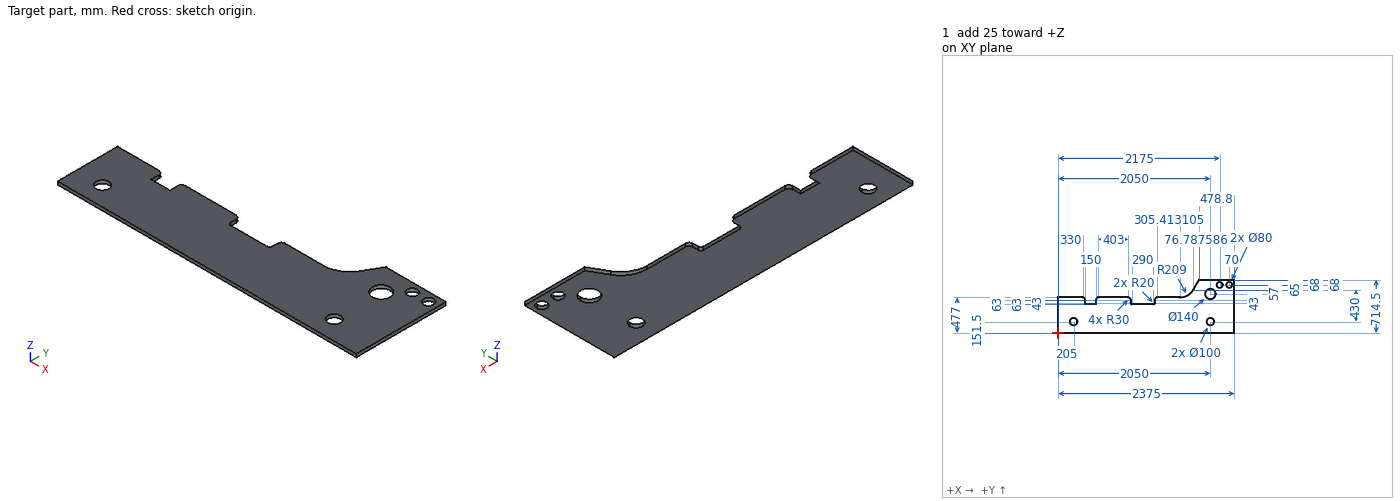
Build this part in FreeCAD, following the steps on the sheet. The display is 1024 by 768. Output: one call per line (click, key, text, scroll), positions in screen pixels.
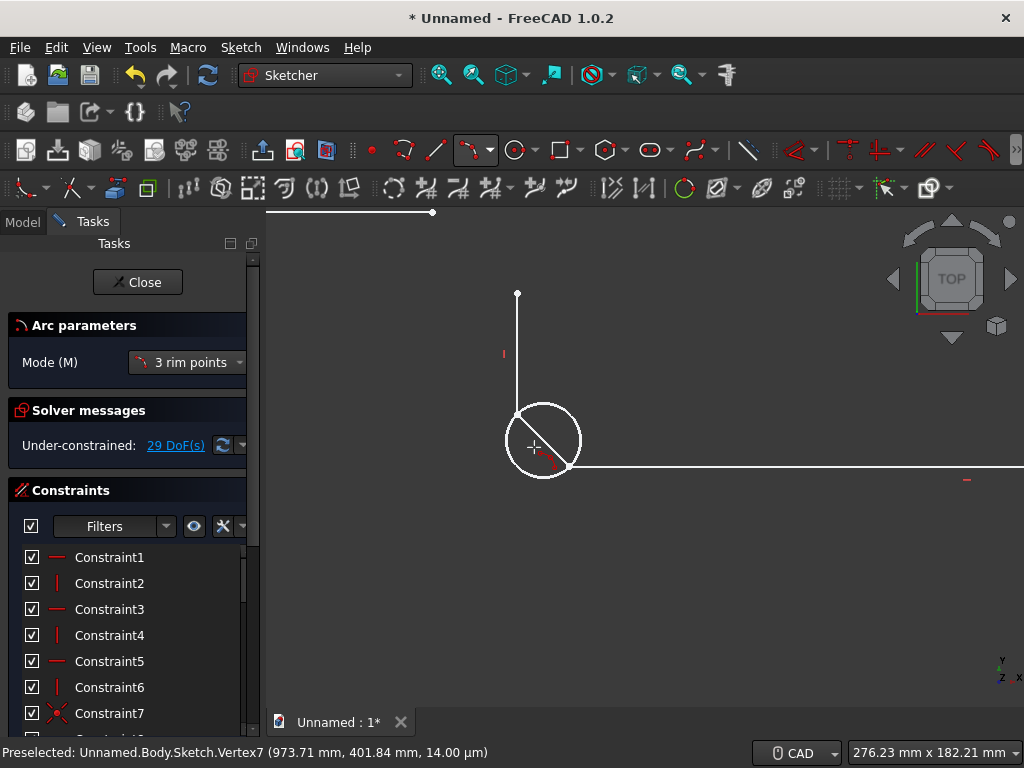
click(531, 447)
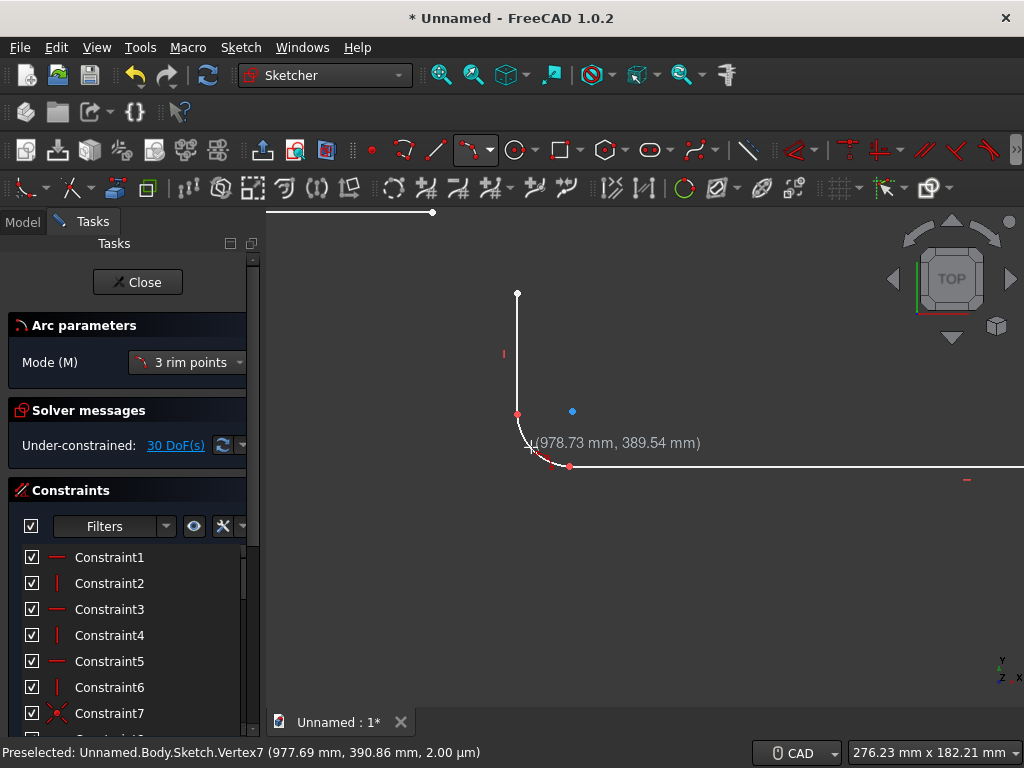
scroll(542, 452, down, 14)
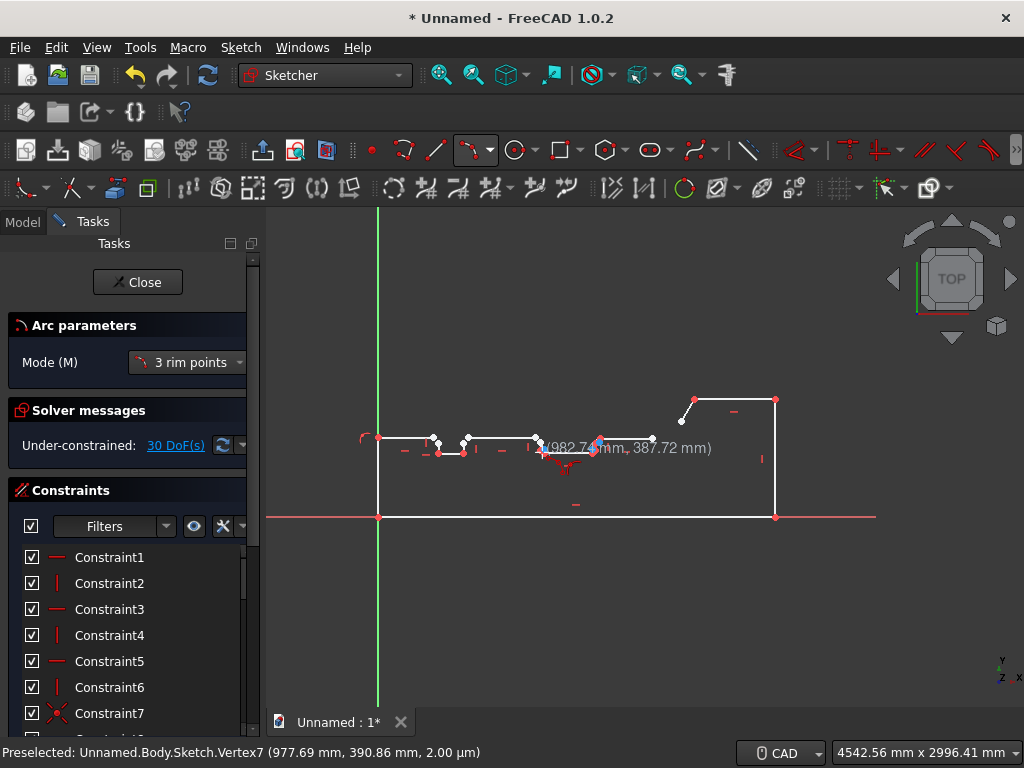
scroll(541, 443, up, 8)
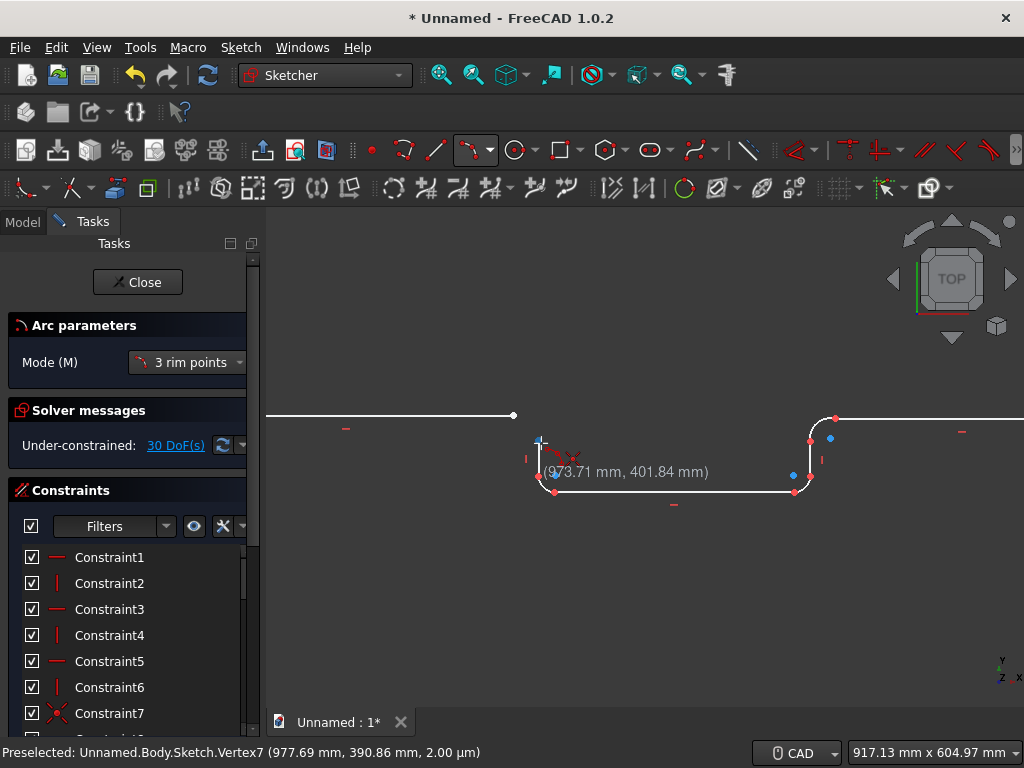
click(539, 440)
click(513, 416)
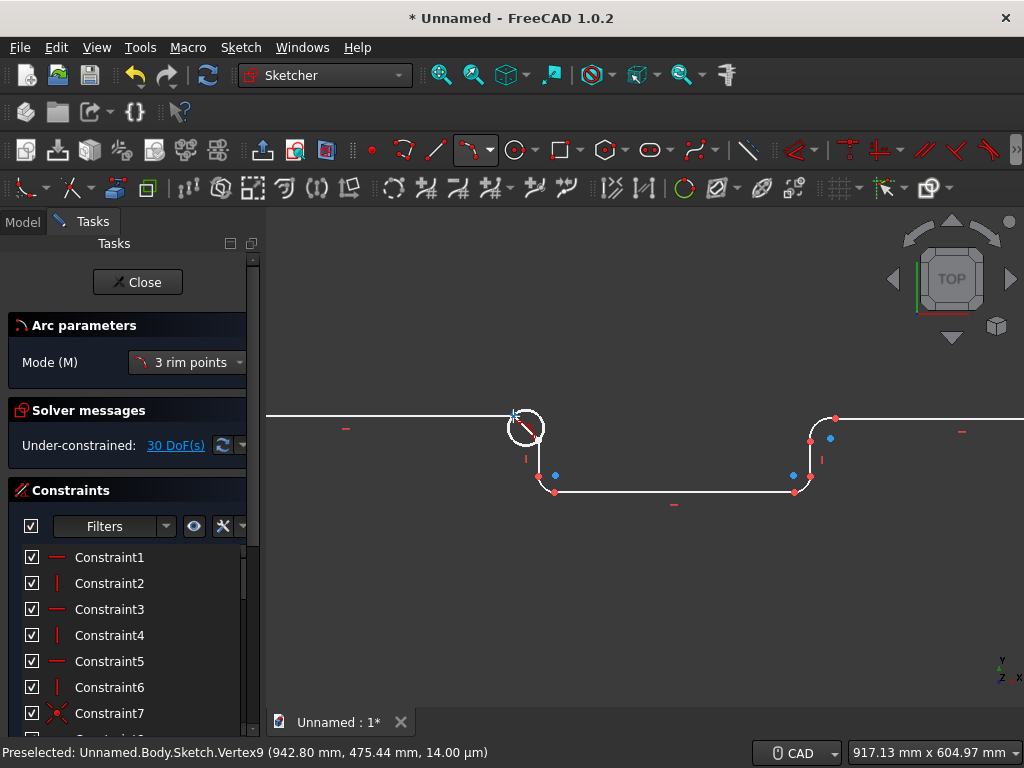
scroll(531, 422, up, 4)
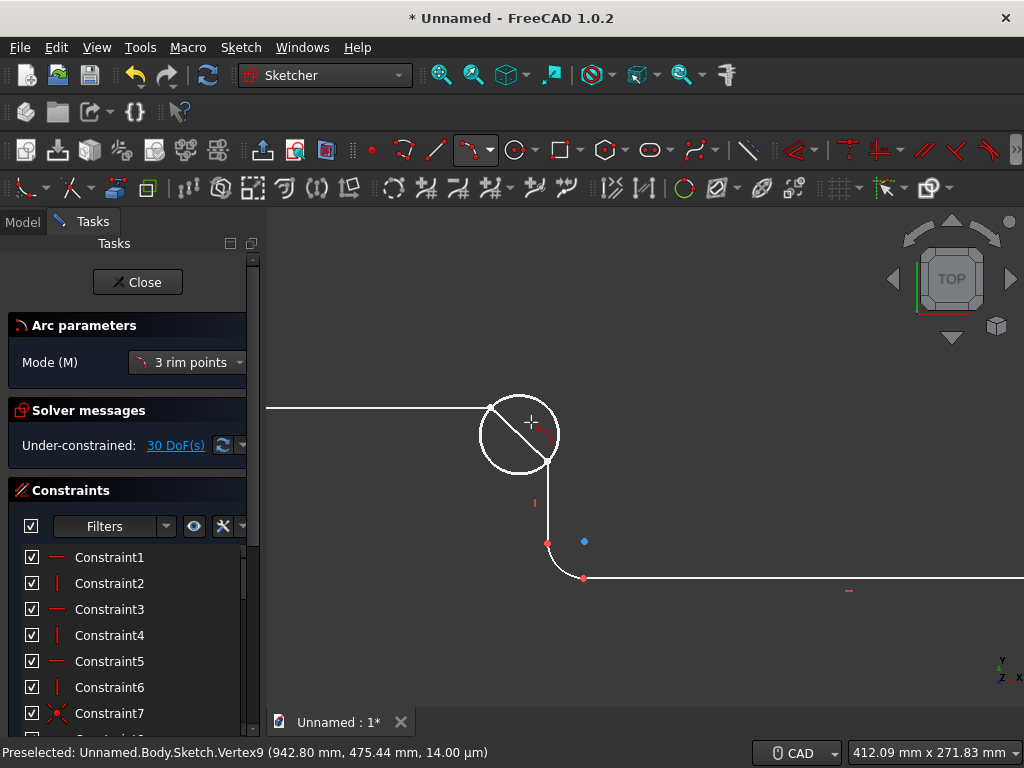
click(530, 421)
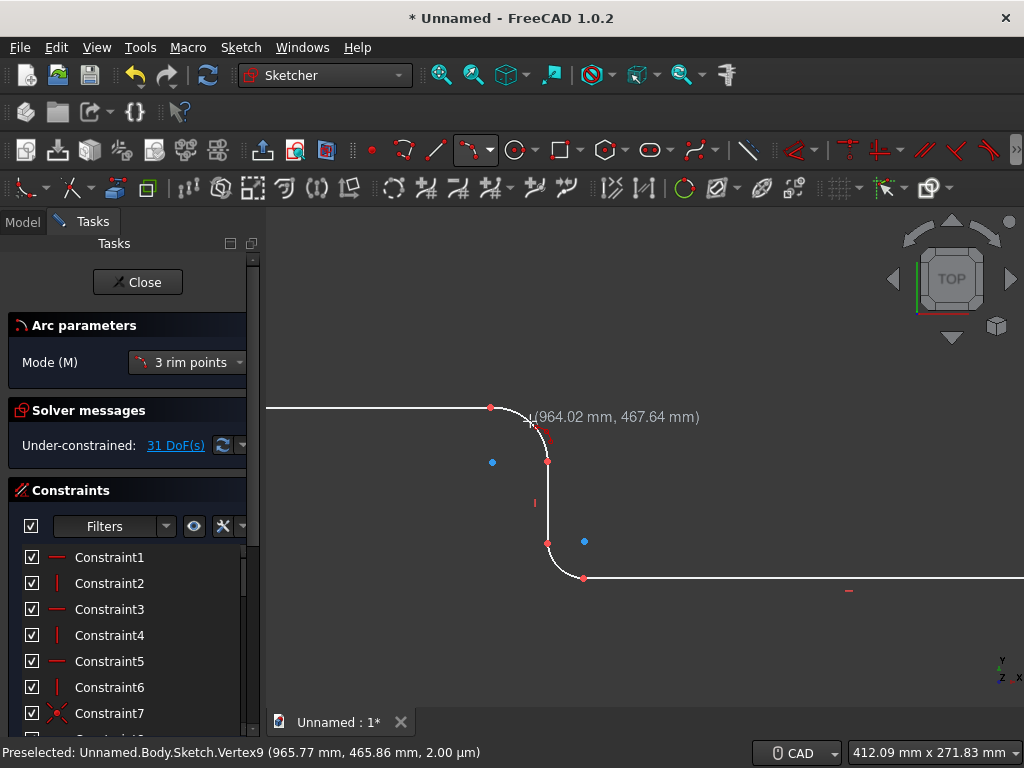
scroll(540, 440, down, 12)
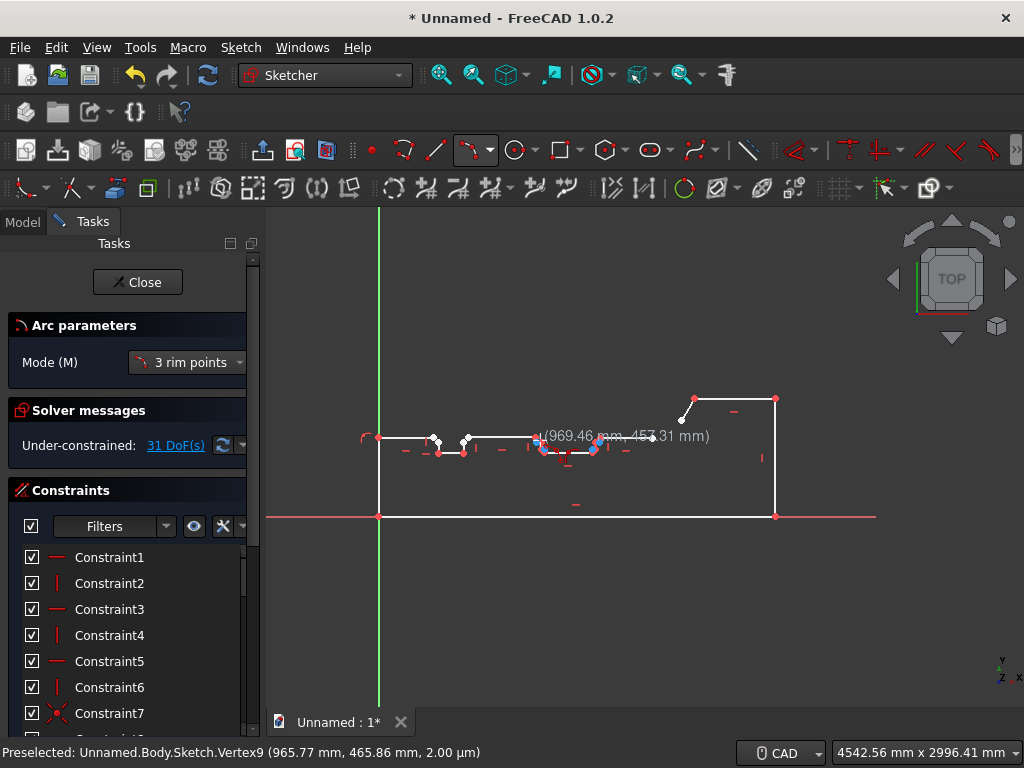
scroll(469, 437, up, 5)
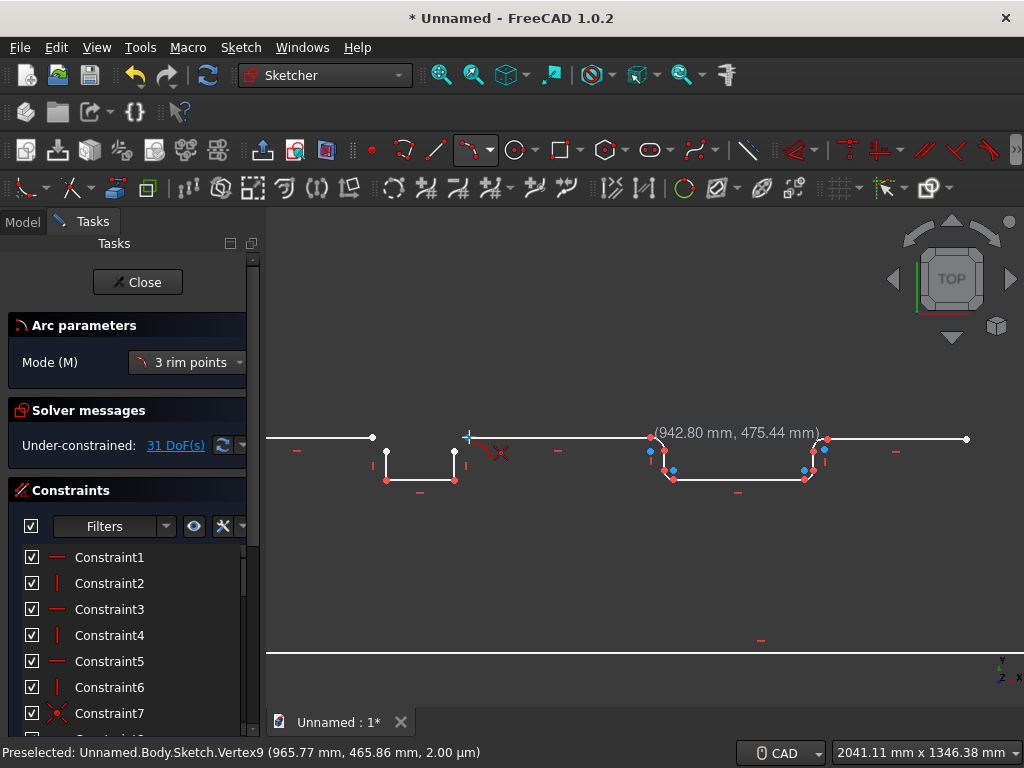
click(467, 438)
click(454, 452)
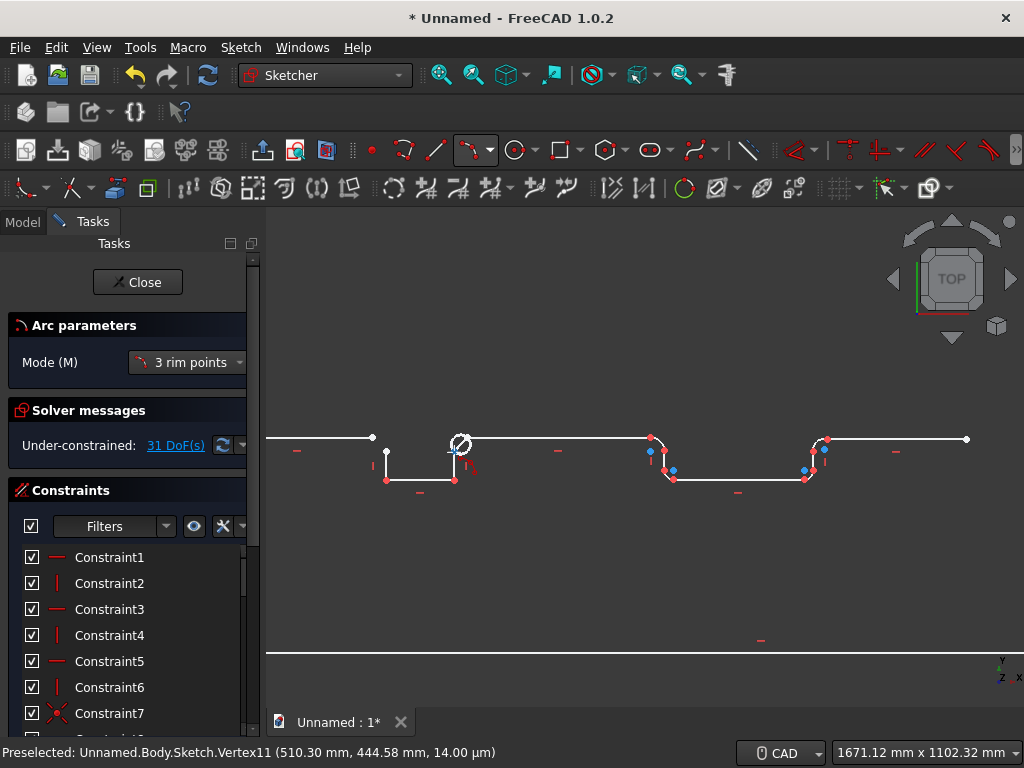
scroll(458, 441, up, 7)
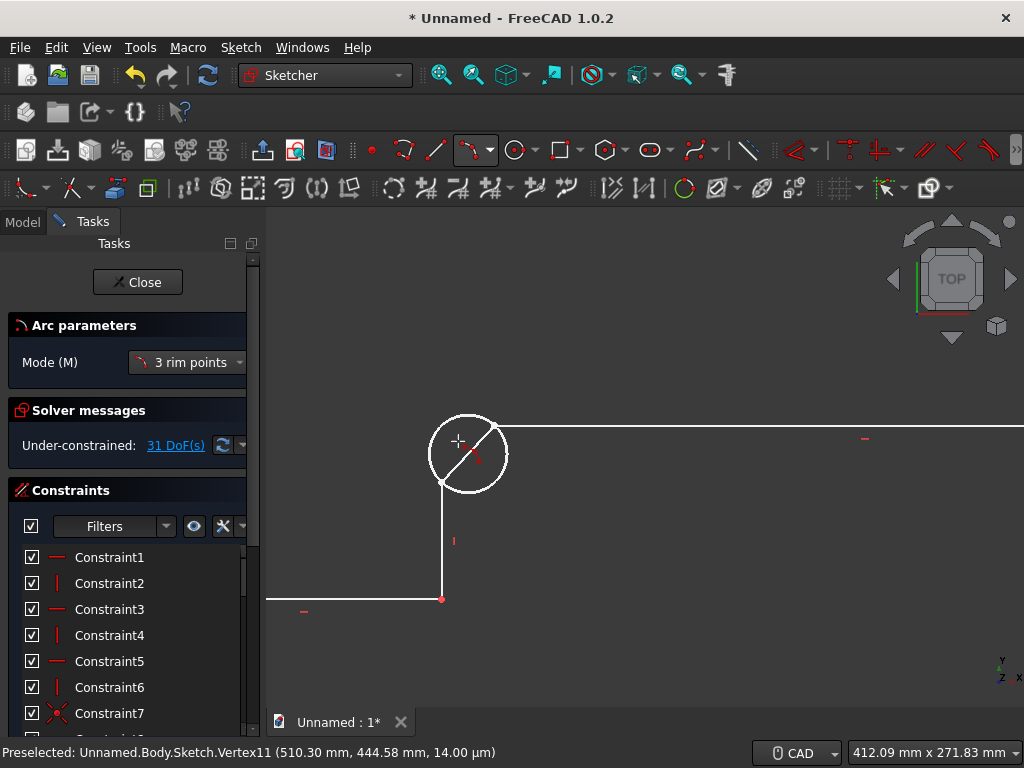
click(457, 439)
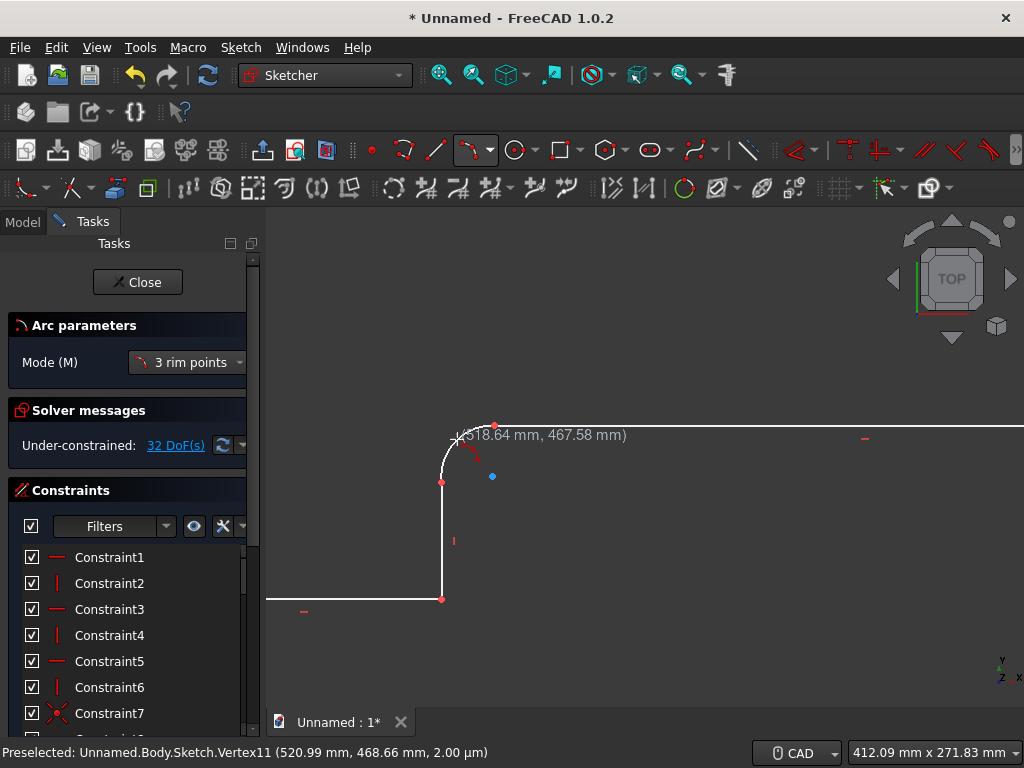
scroll(466, 438, down, 12)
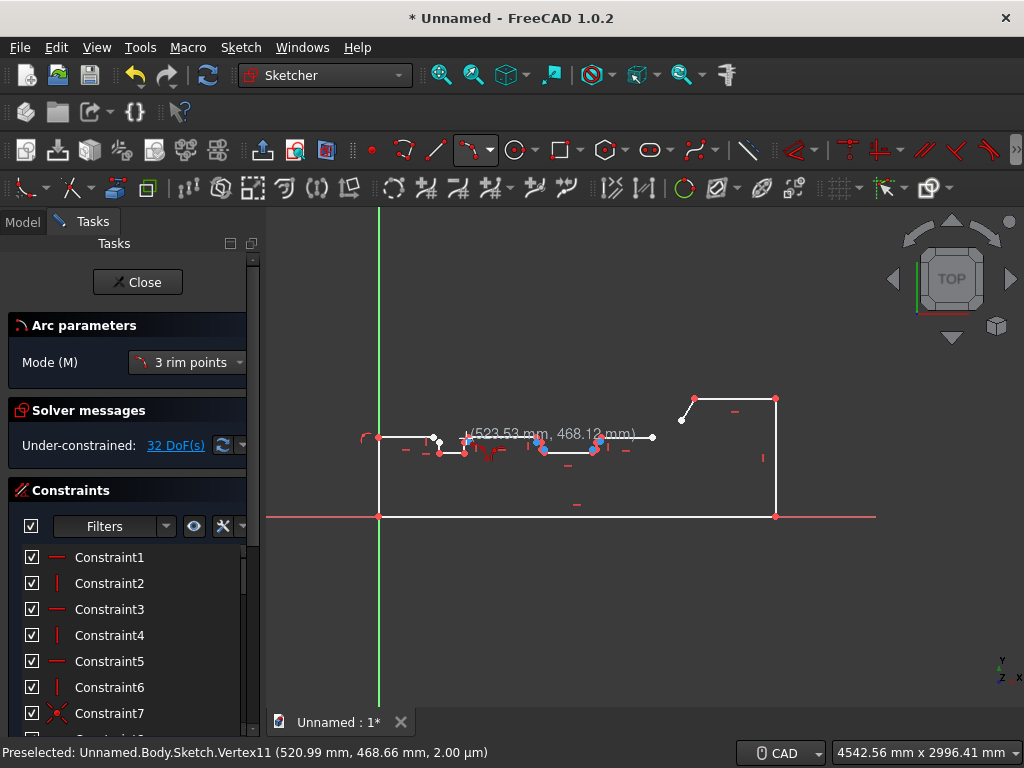
scroll(439, 442, up, 6)